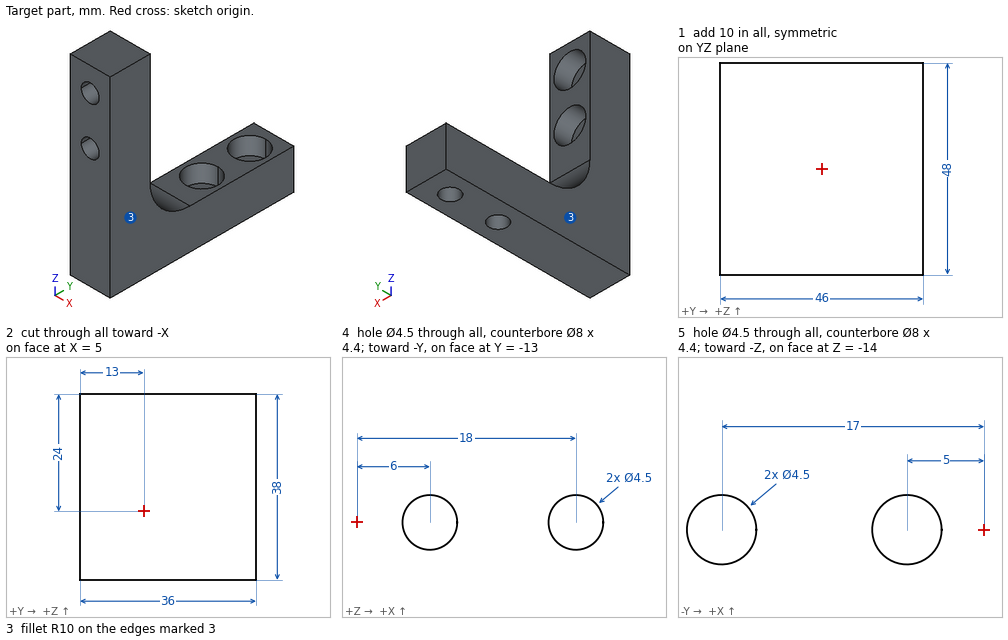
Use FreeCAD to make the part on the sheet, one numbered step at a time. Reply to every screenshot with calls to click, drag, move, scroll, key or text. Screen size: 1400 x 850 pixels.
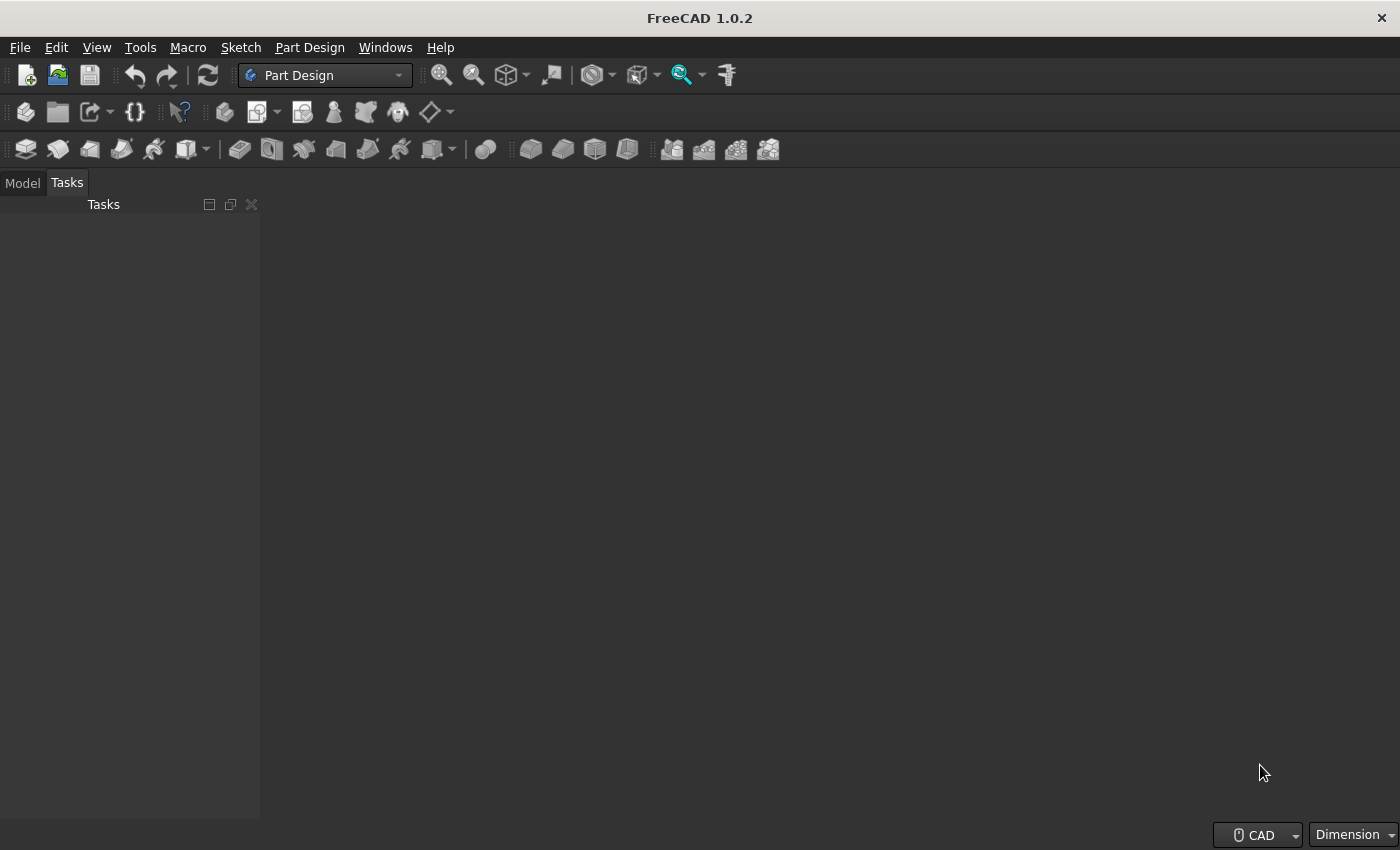
click(26, 76)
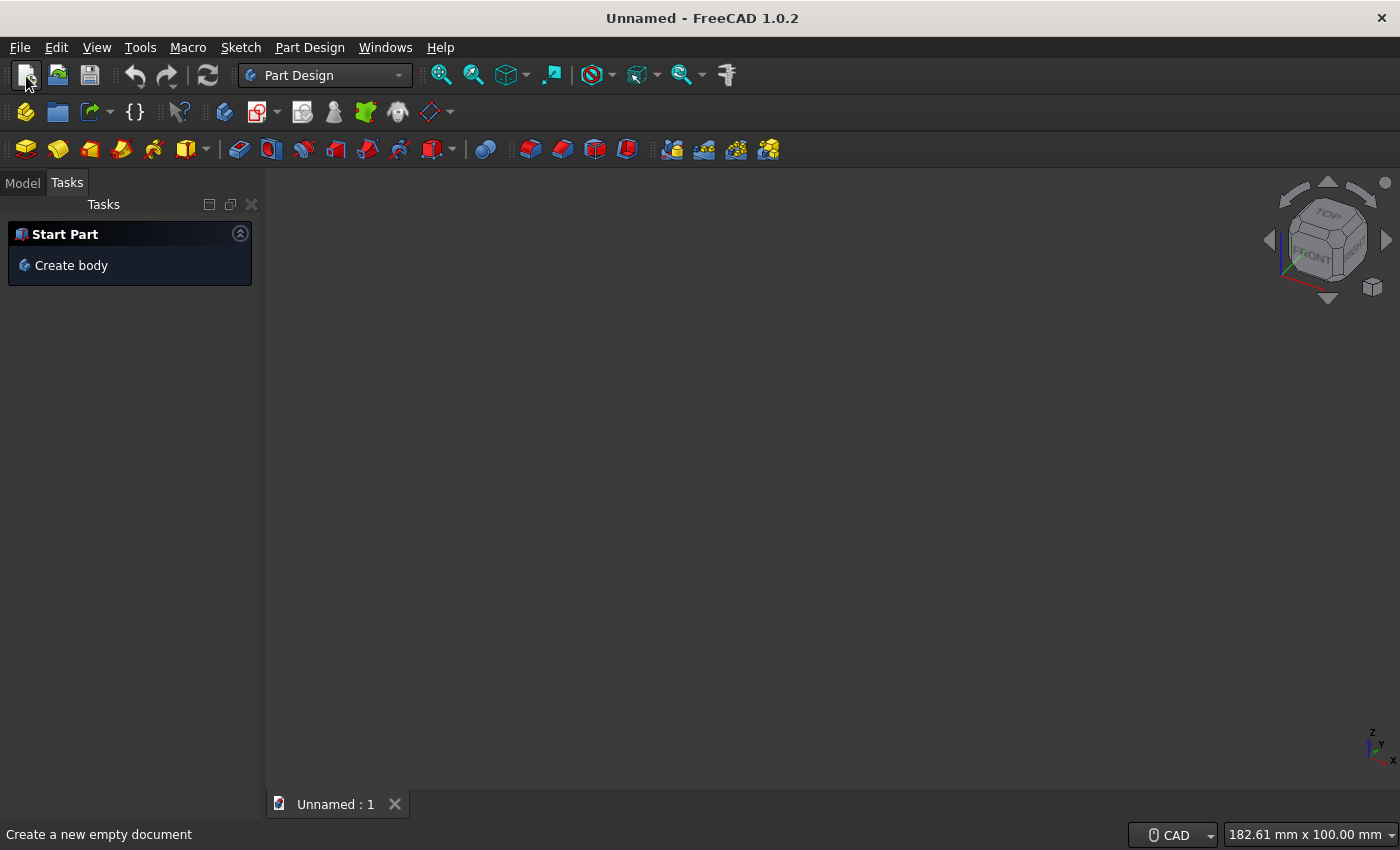
click(258, 112)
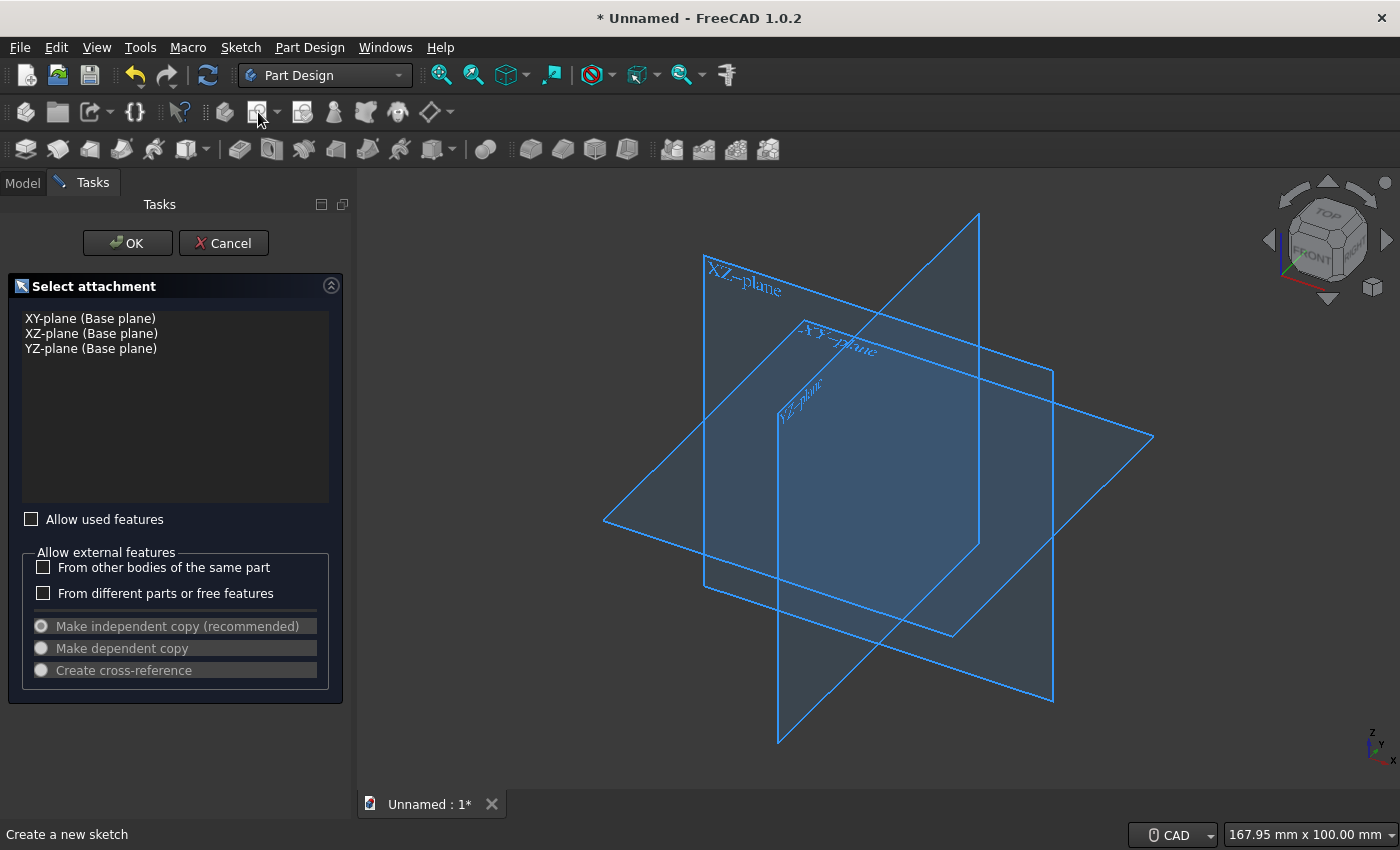
click(82, 348)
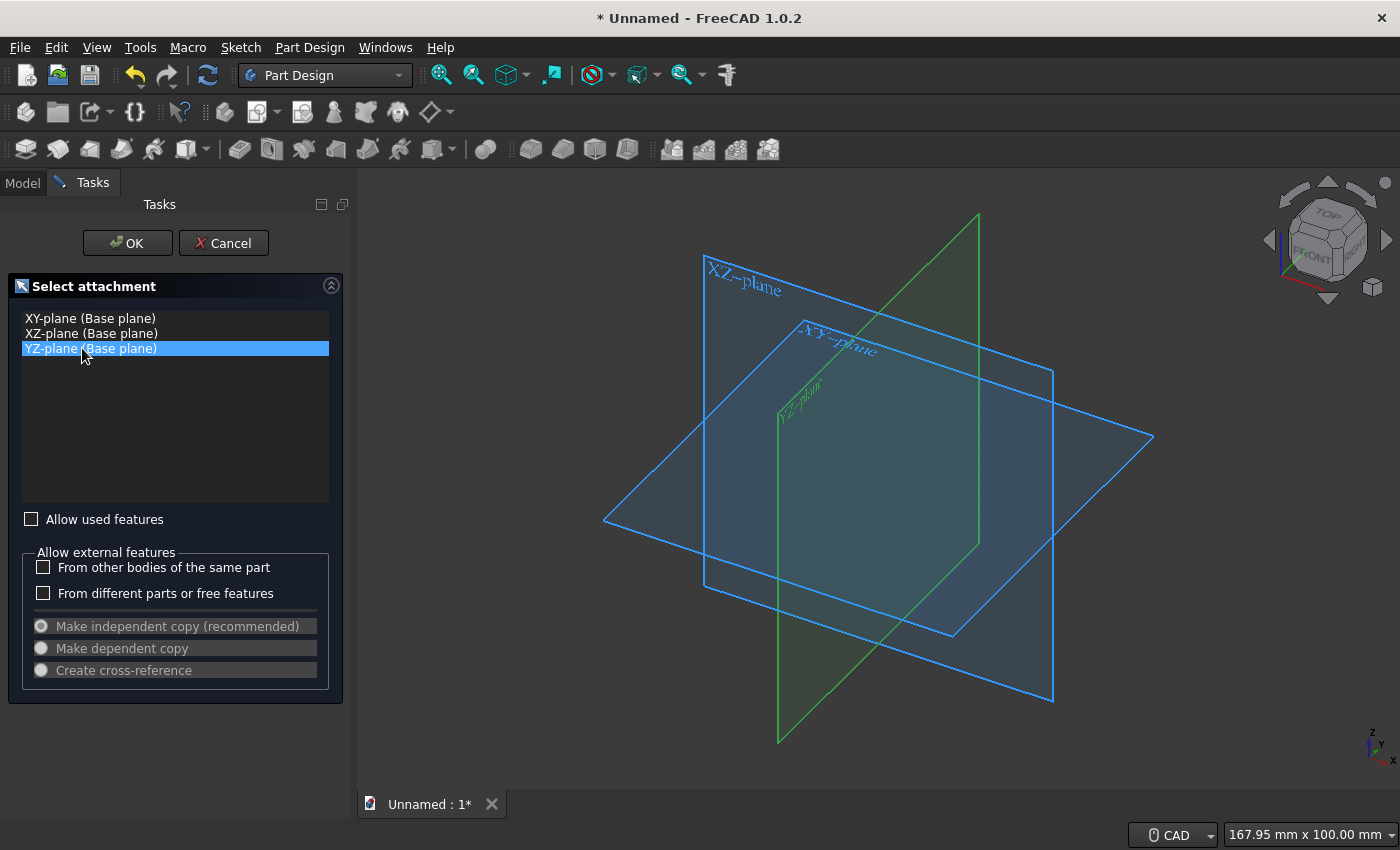
click(128, 243)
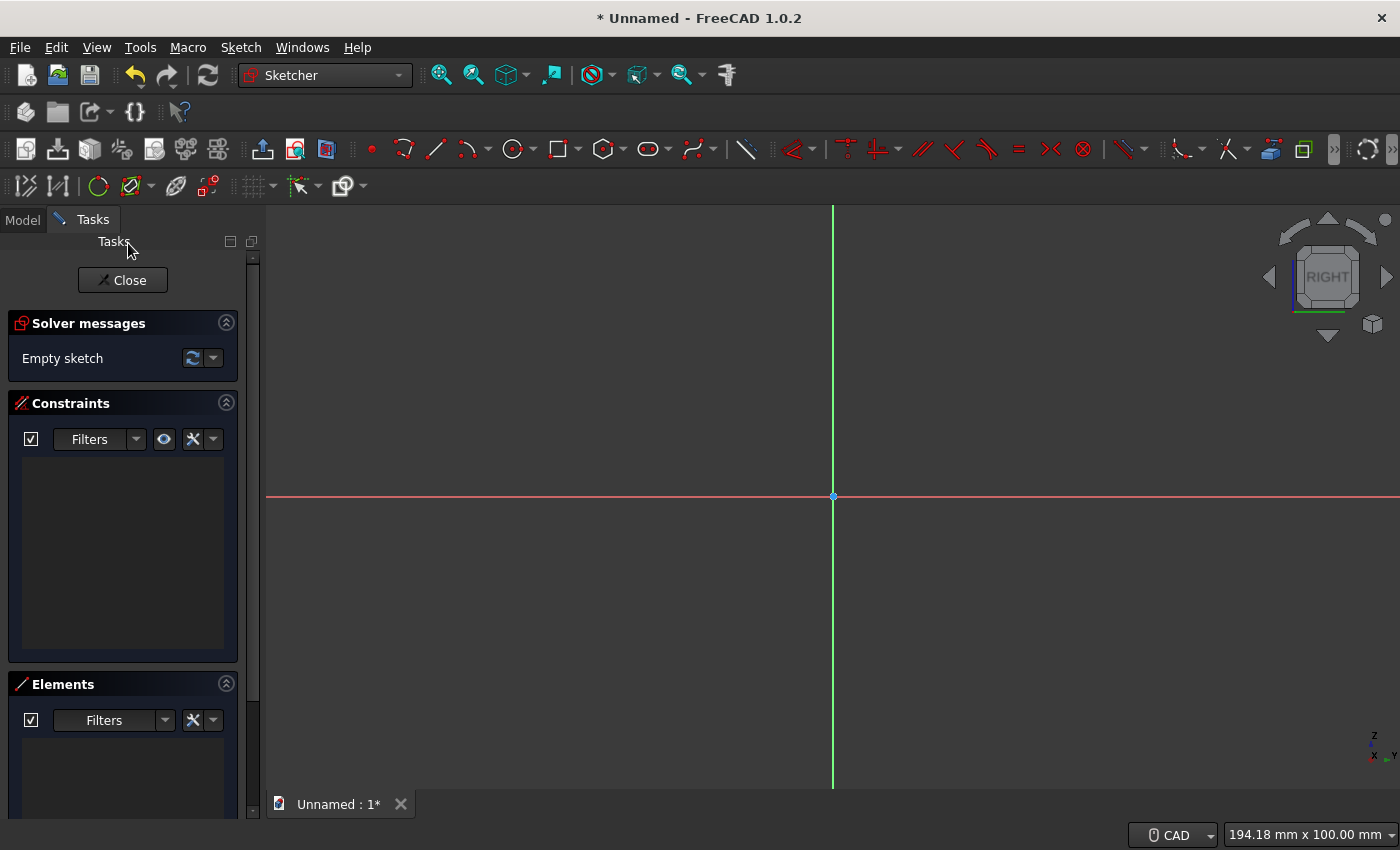
click(580, 150)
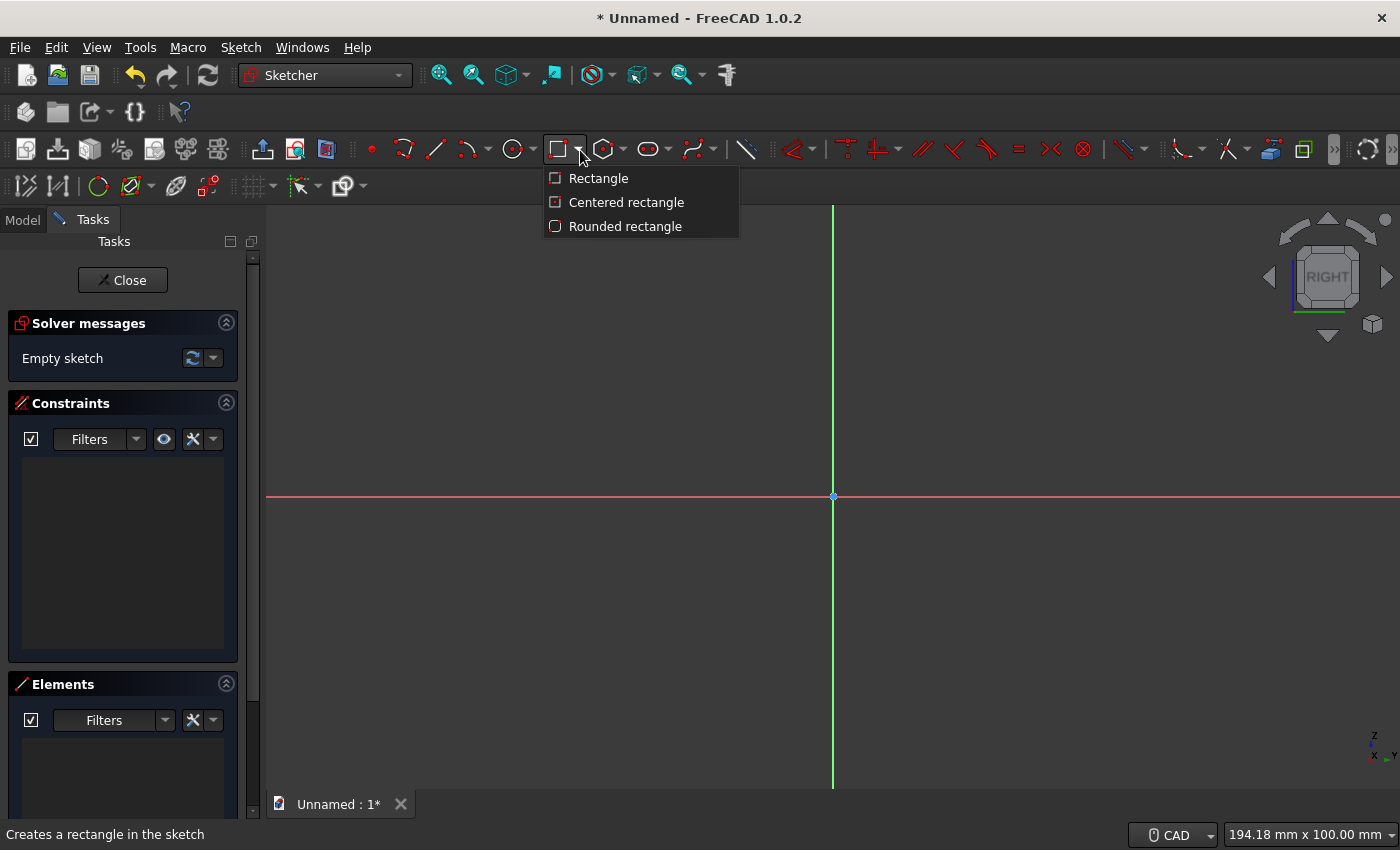
click(642, 202)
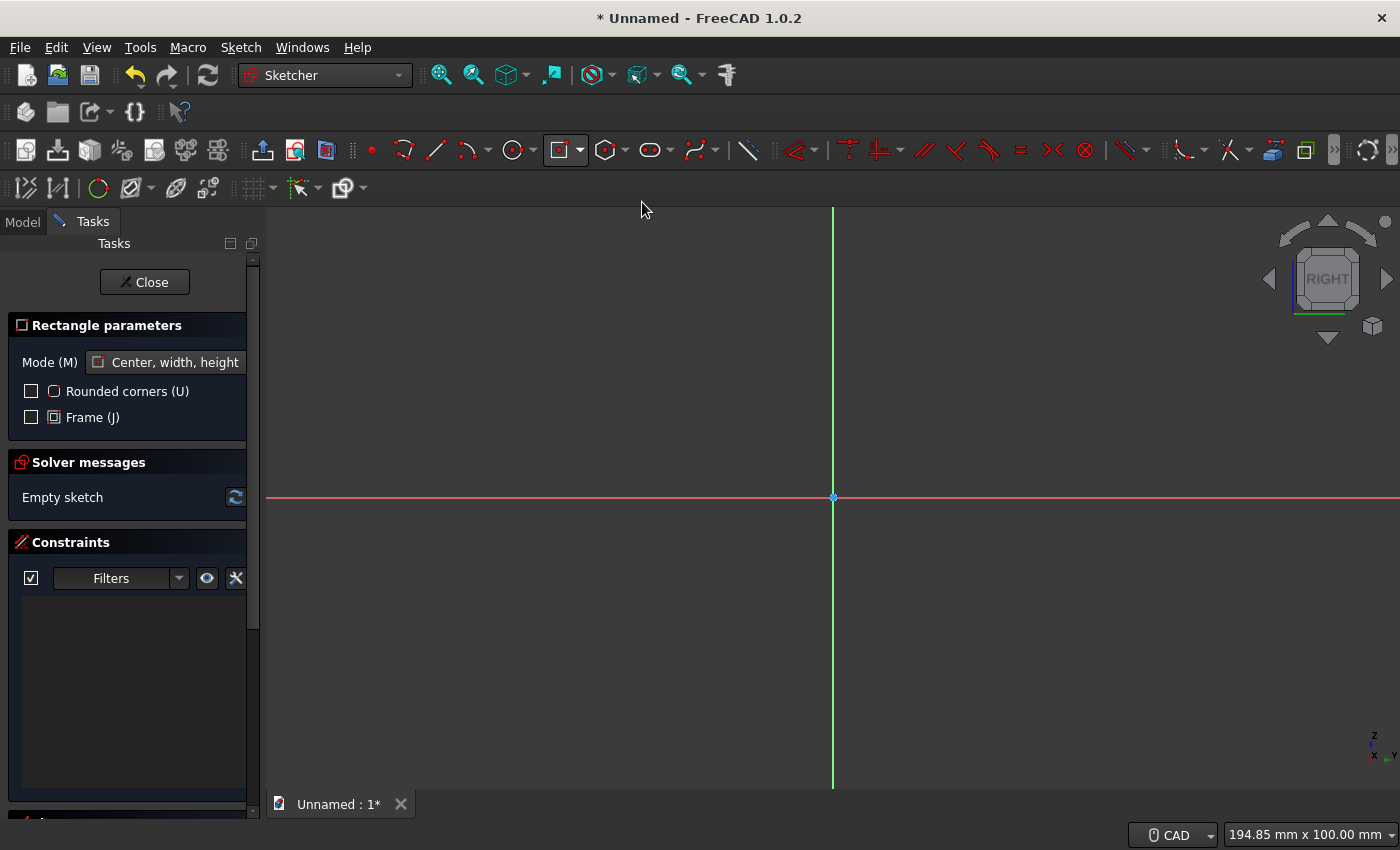
click(833, 498)
move(967, 358)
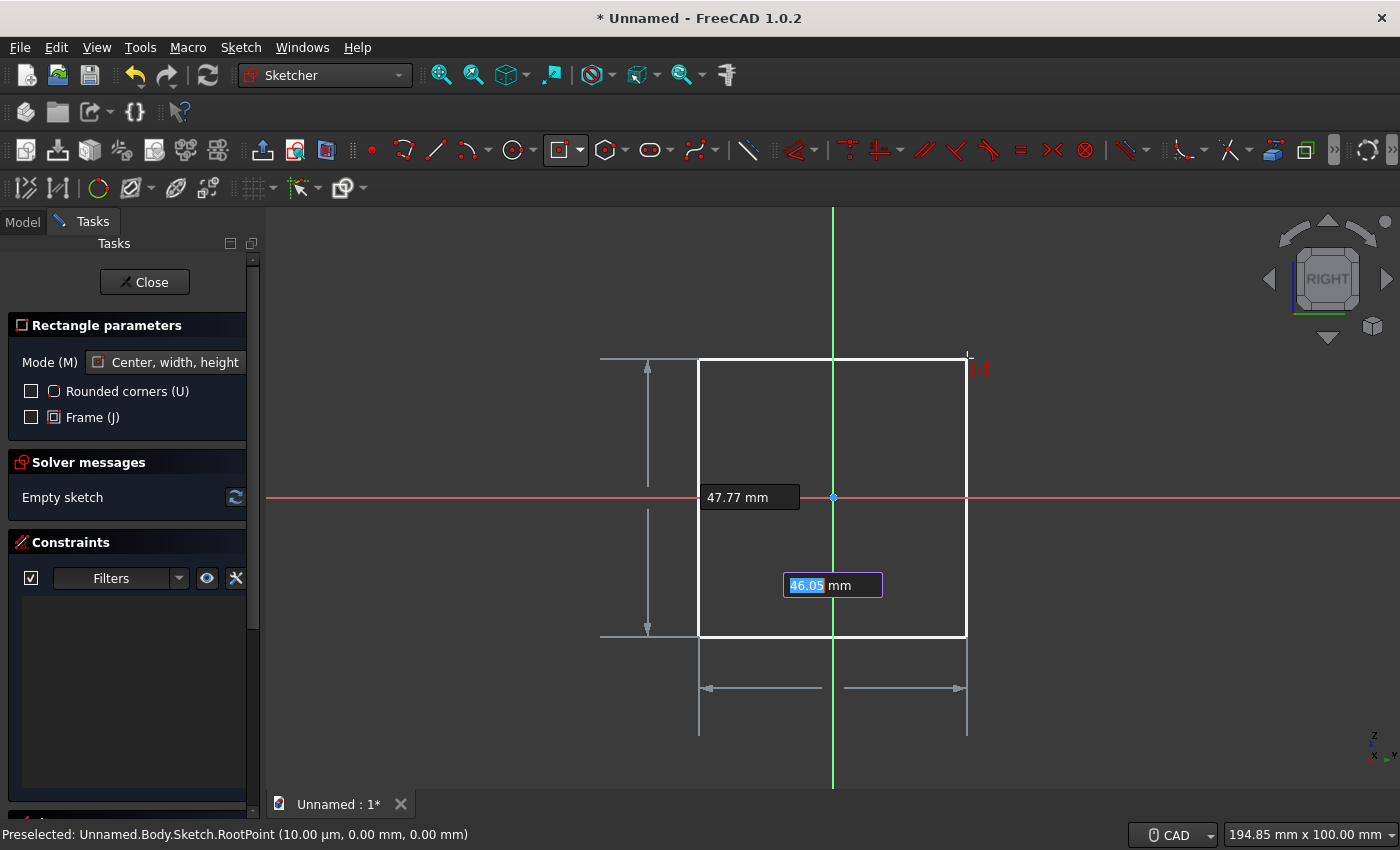
text(46)
key(Tab)
text(48)
key(Return)
key(Escape)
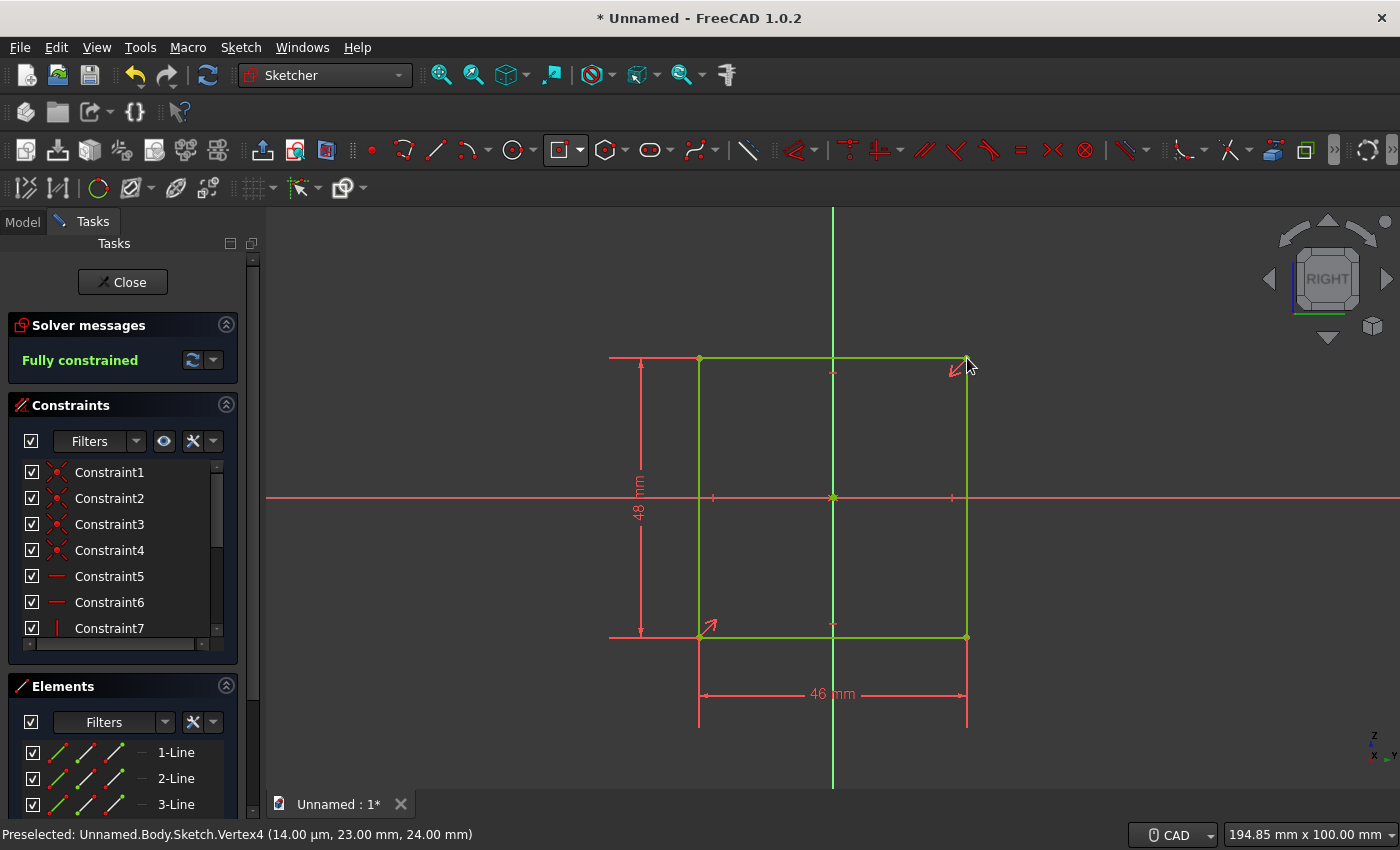
click(123, 282)